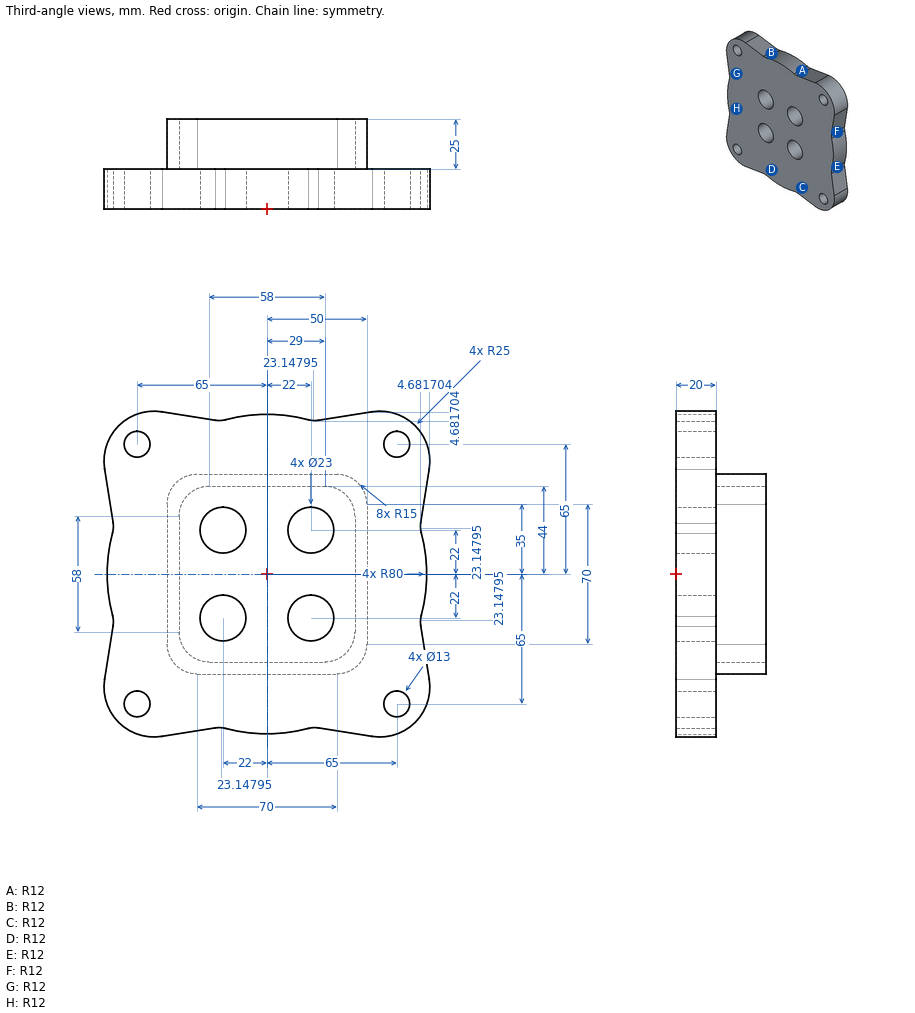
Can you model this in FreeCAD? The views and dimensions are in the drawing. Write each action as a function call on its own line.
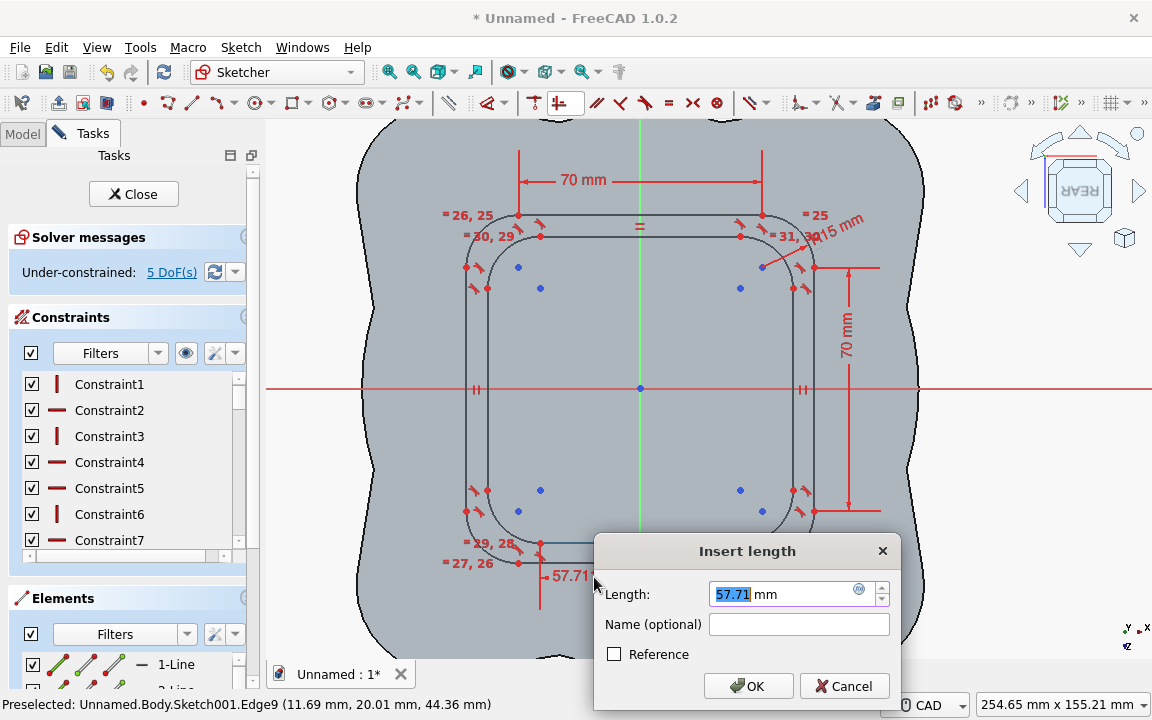
text(58)
key(Return)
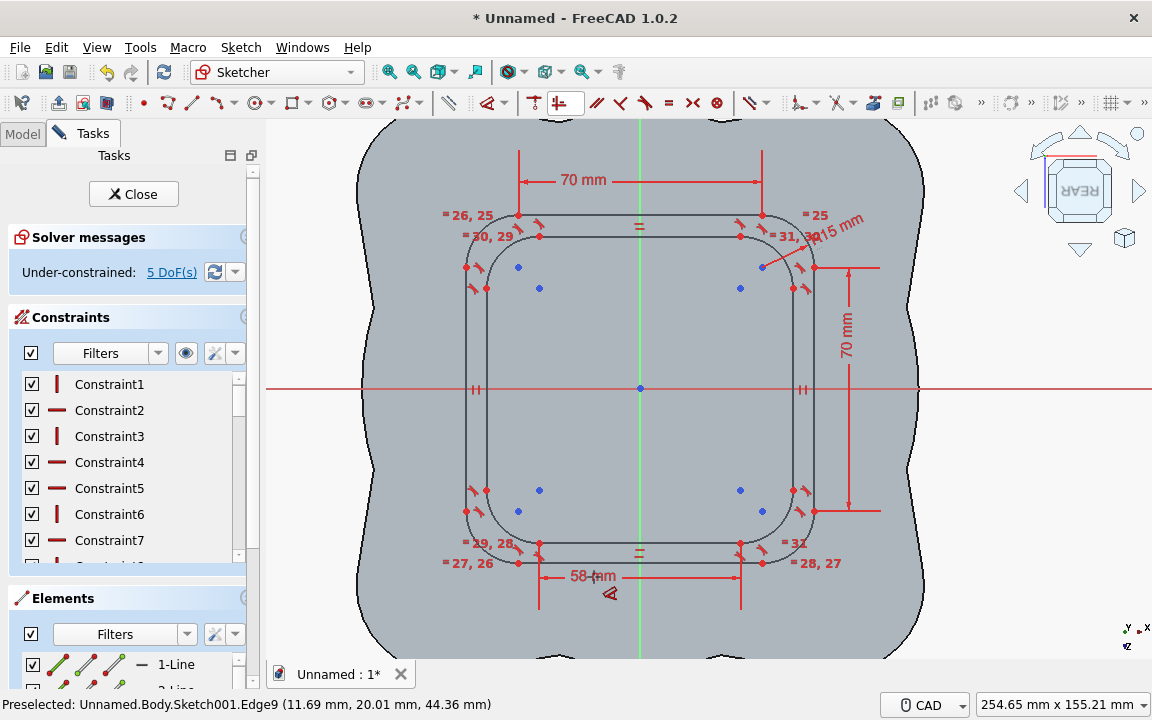
click(487, 430)
click(453, 343)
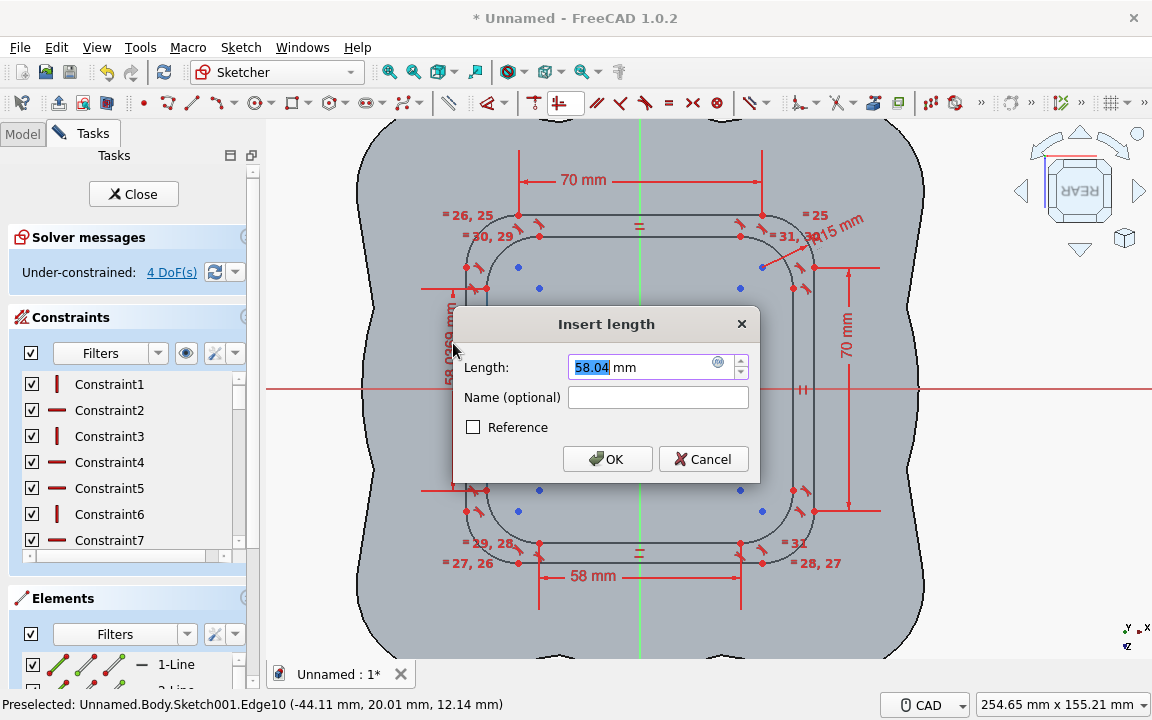
text(58)
key(Return)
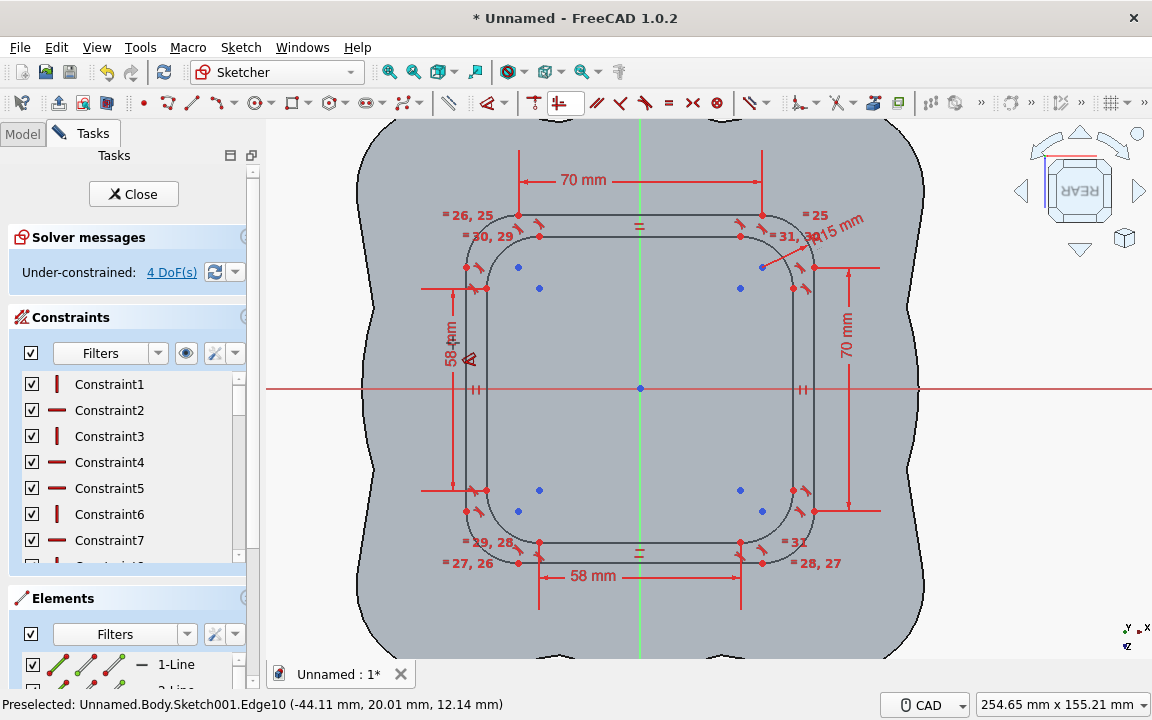
click(814, 511)
click(727, 355)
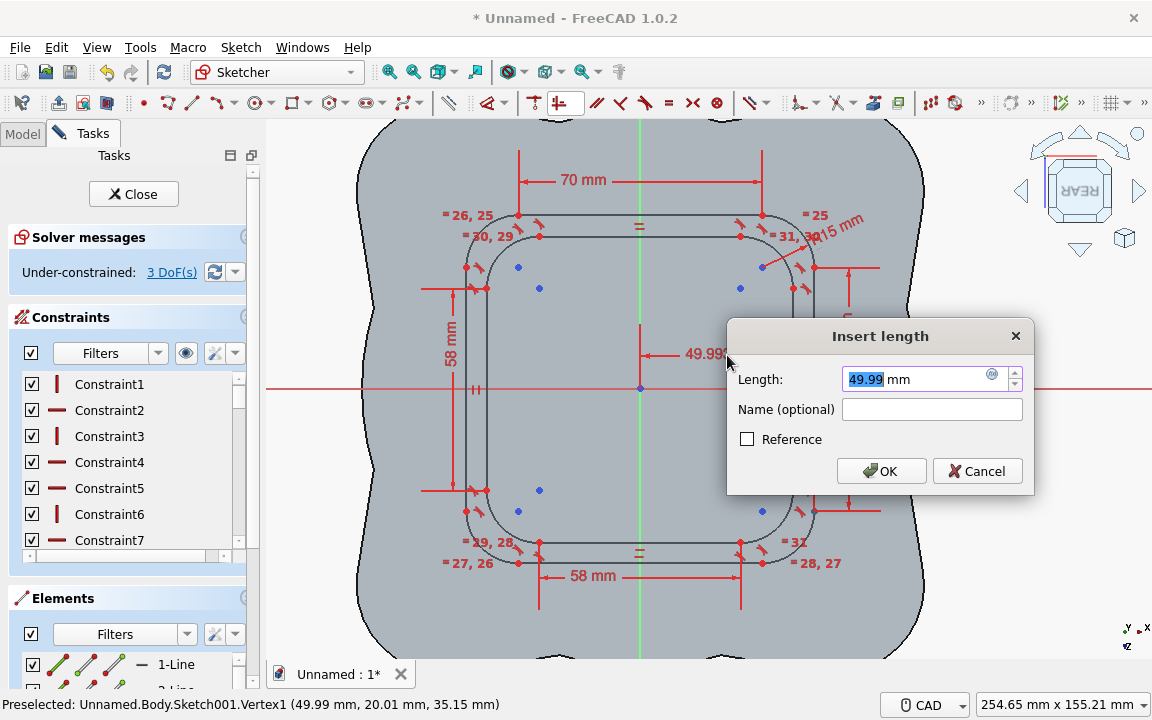
text(50)
key(Return)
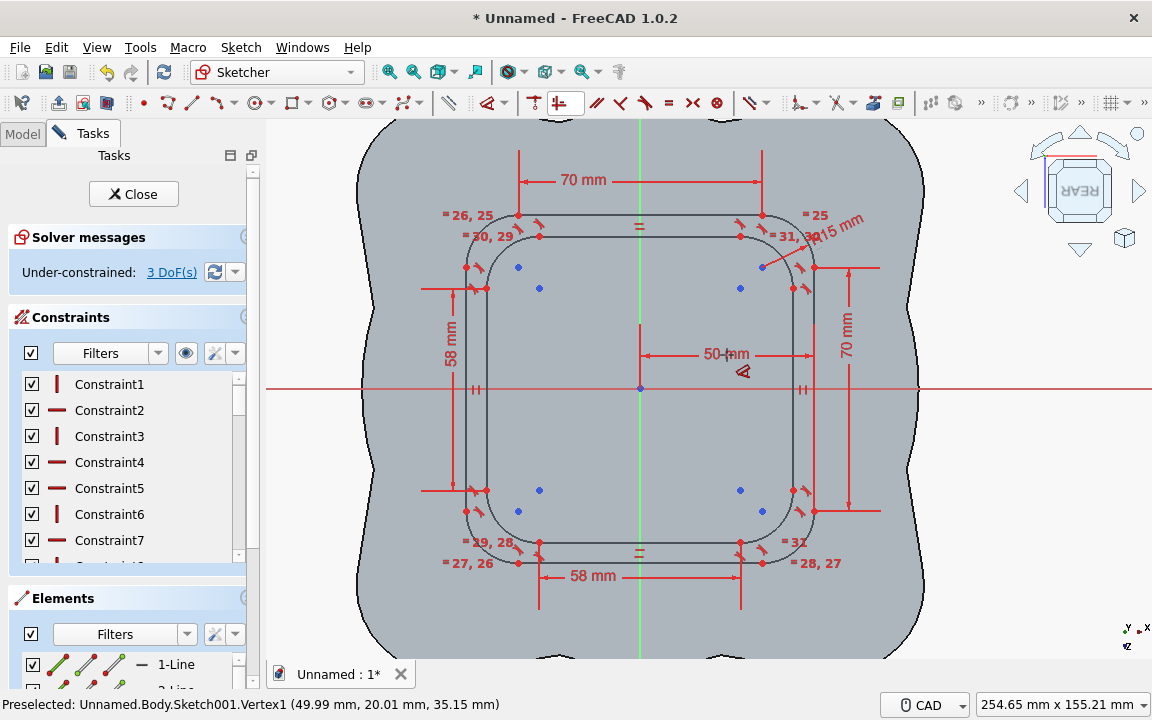
click(814, 511)
click(848, 450)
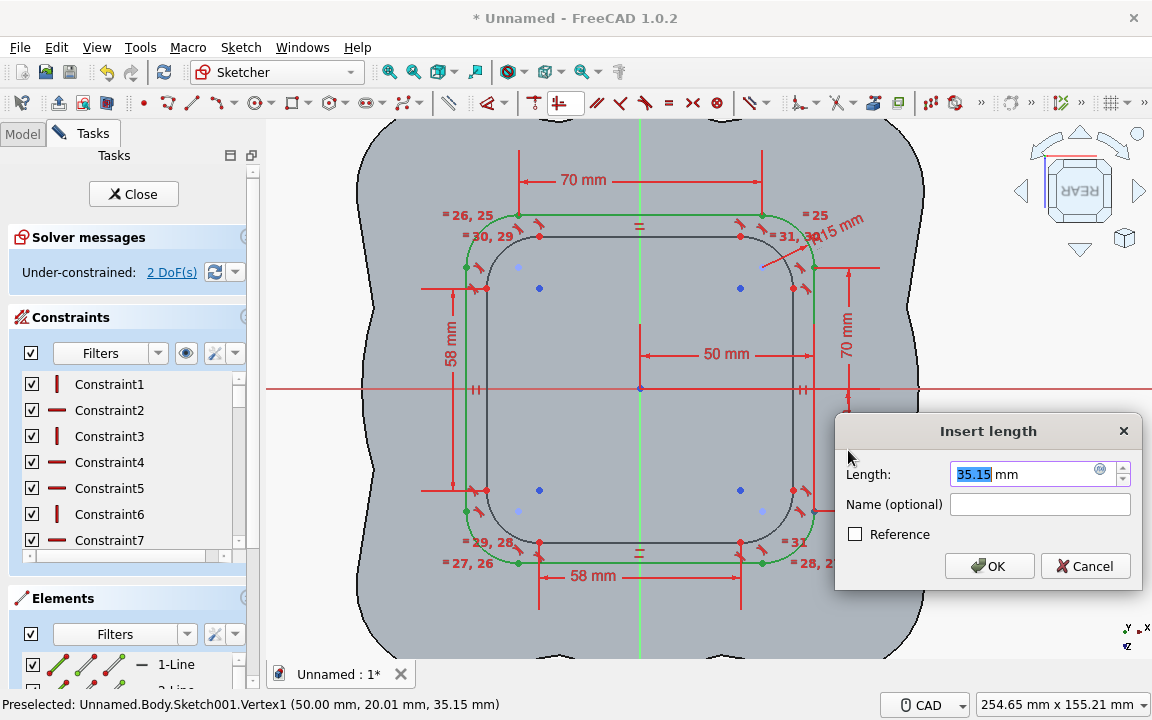
text(35)
key(Return)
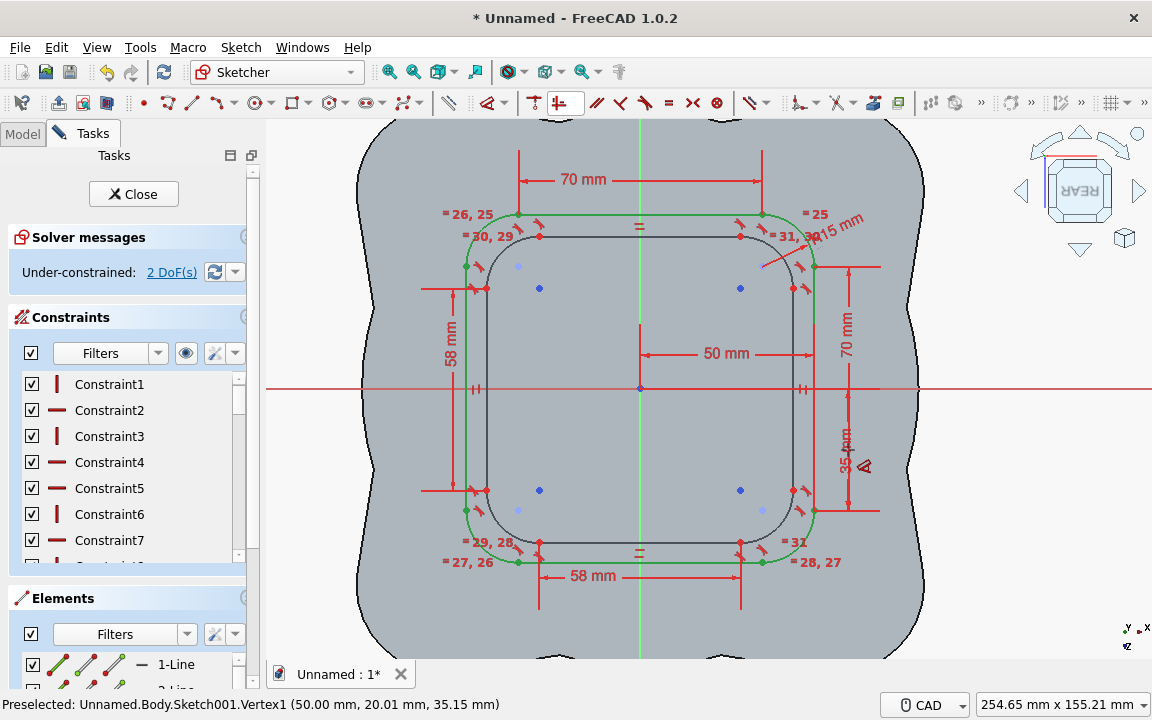
click(741, 543)
click(691, 577)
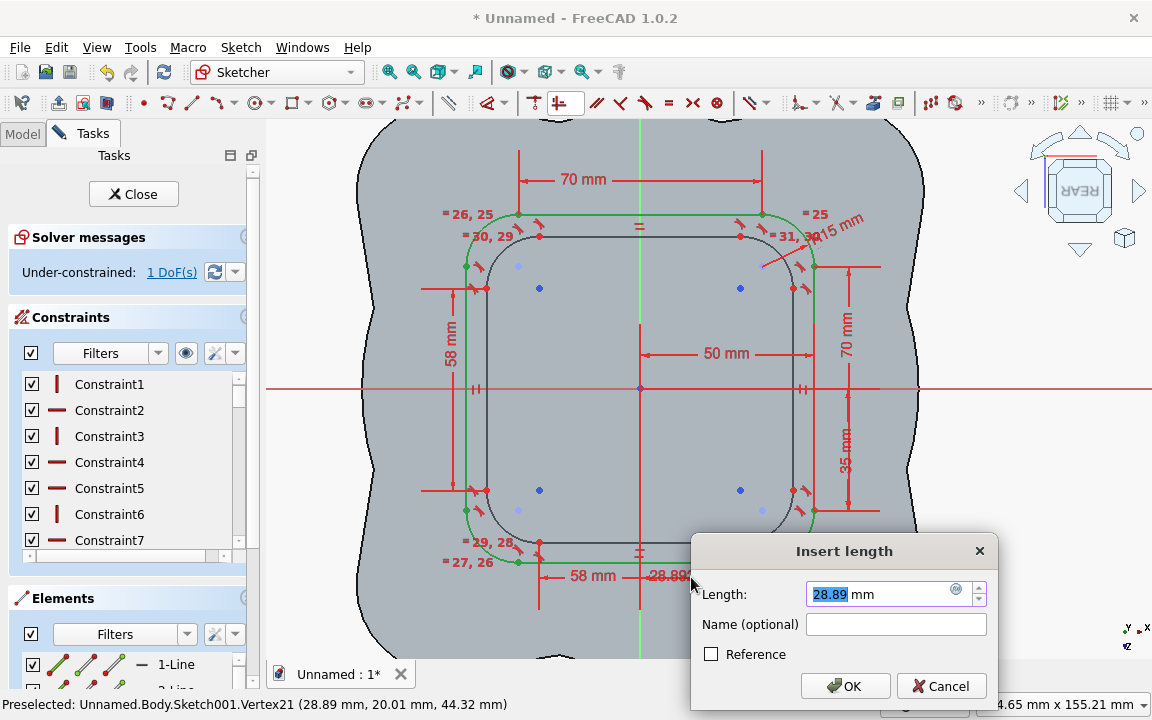
text(29)
key(Return)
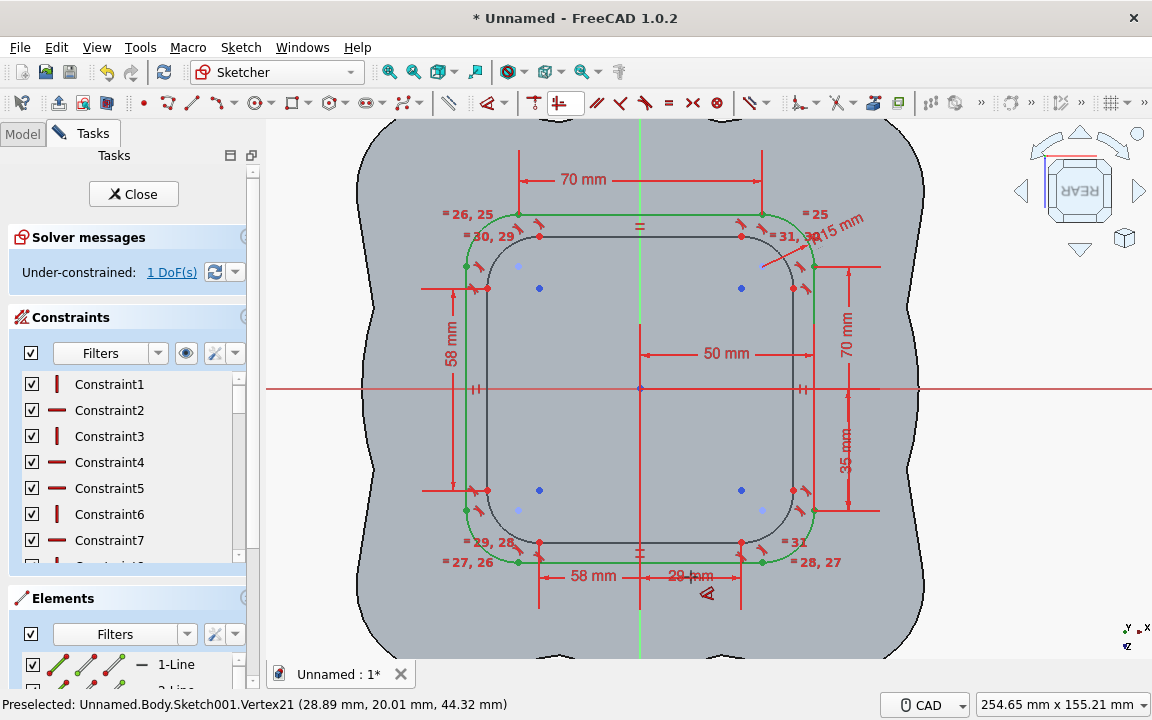
click(741, 543)
click(775, 466)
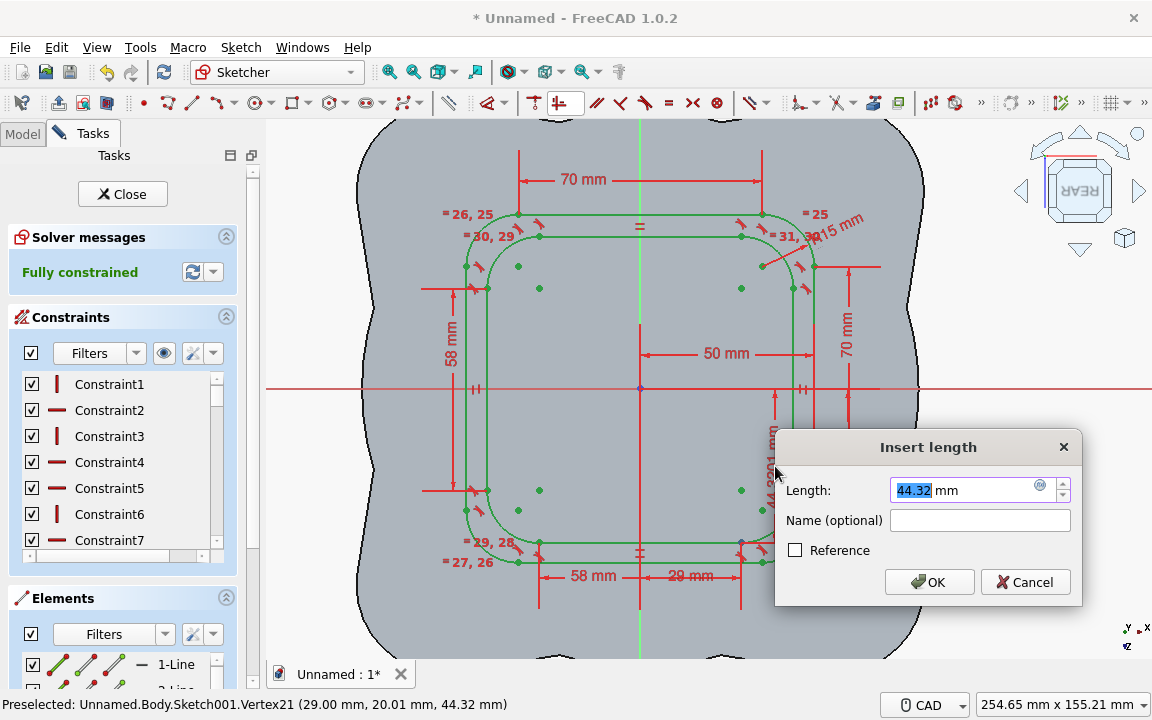
text(44)
key(Return)
key(Escape)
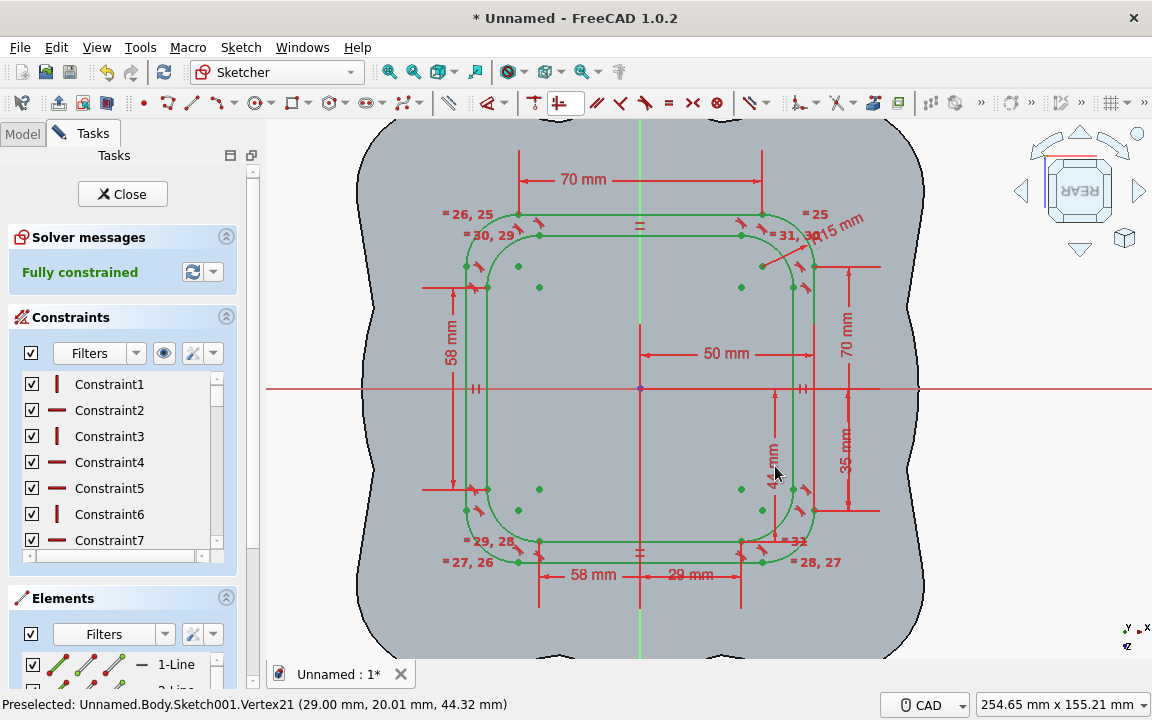
click(123, 194)